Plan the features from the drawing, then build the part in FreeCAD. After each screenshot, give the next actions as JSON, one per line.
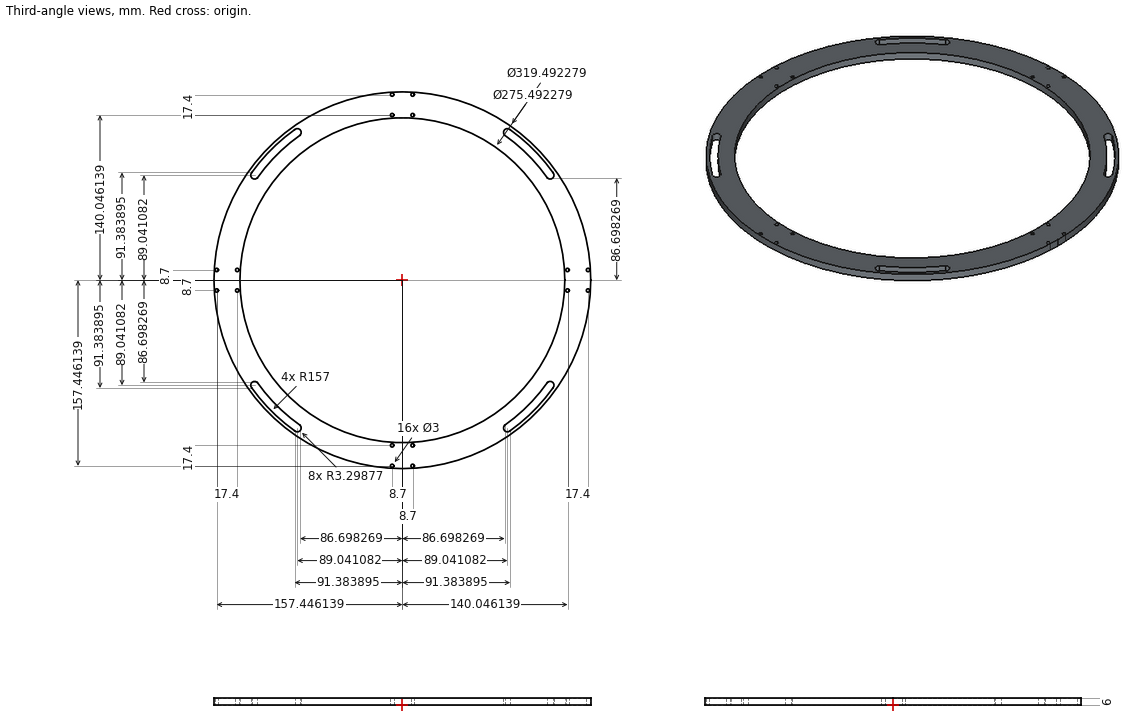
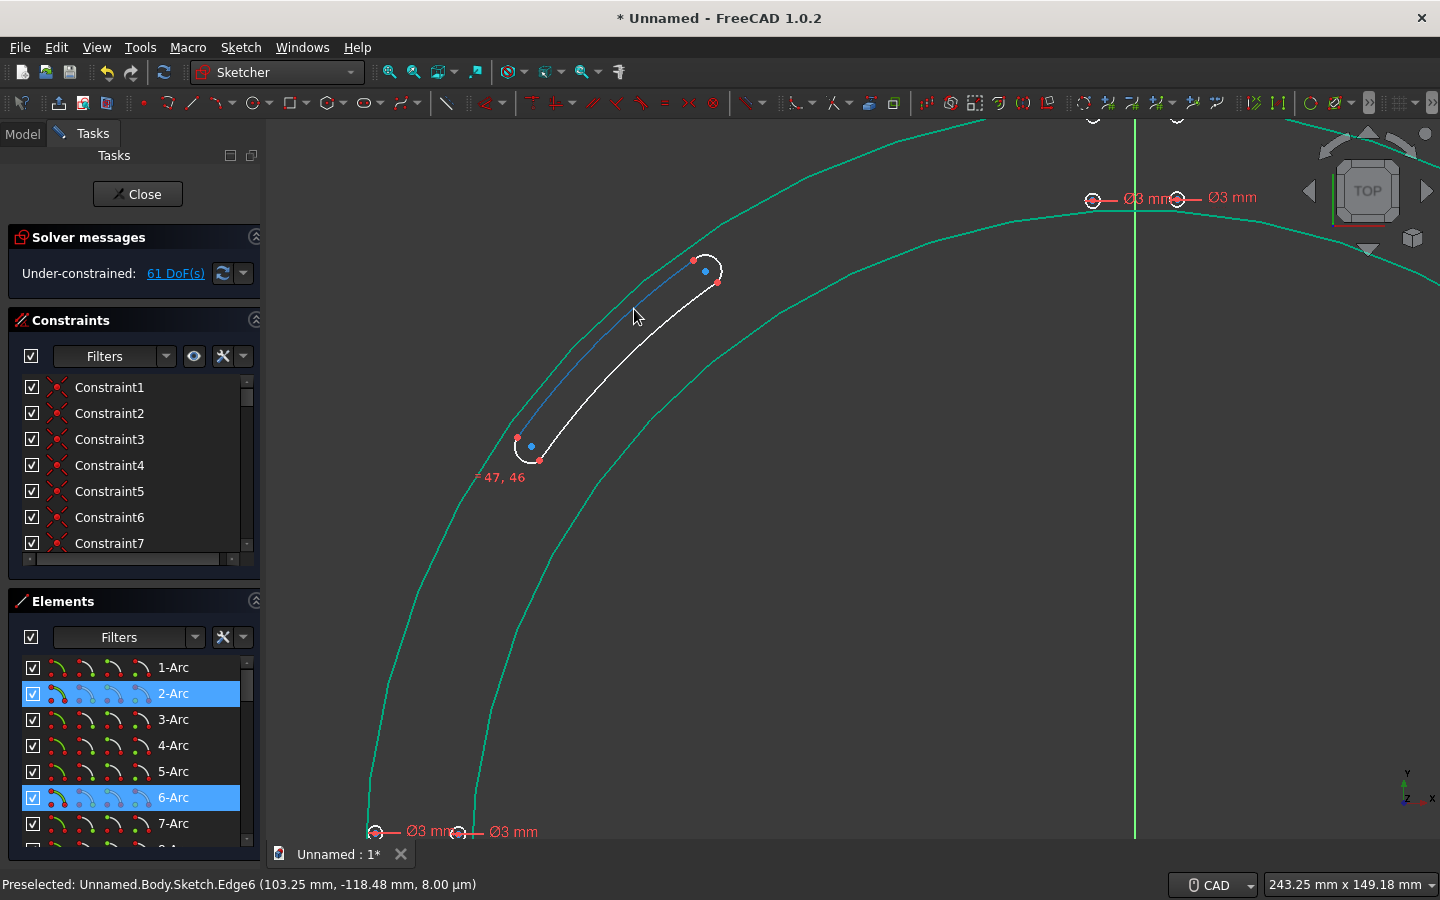
{"action": "left_click", "coordinate": [635, 307]}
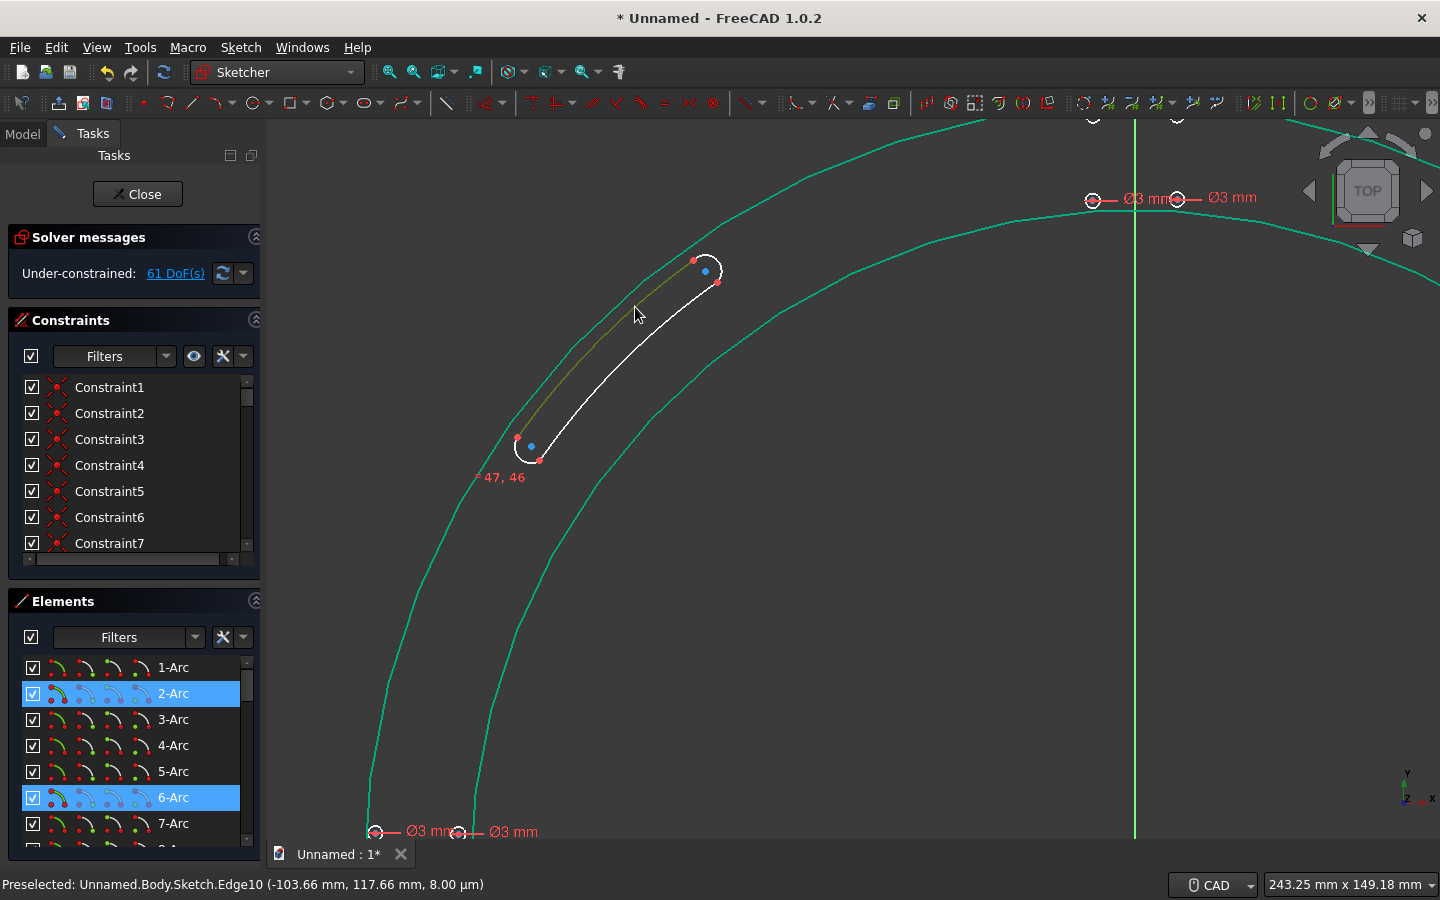
{"action": "scroll", "coordinate": [633, 308], "scroll_direction": "down", "scroll_amount": 6}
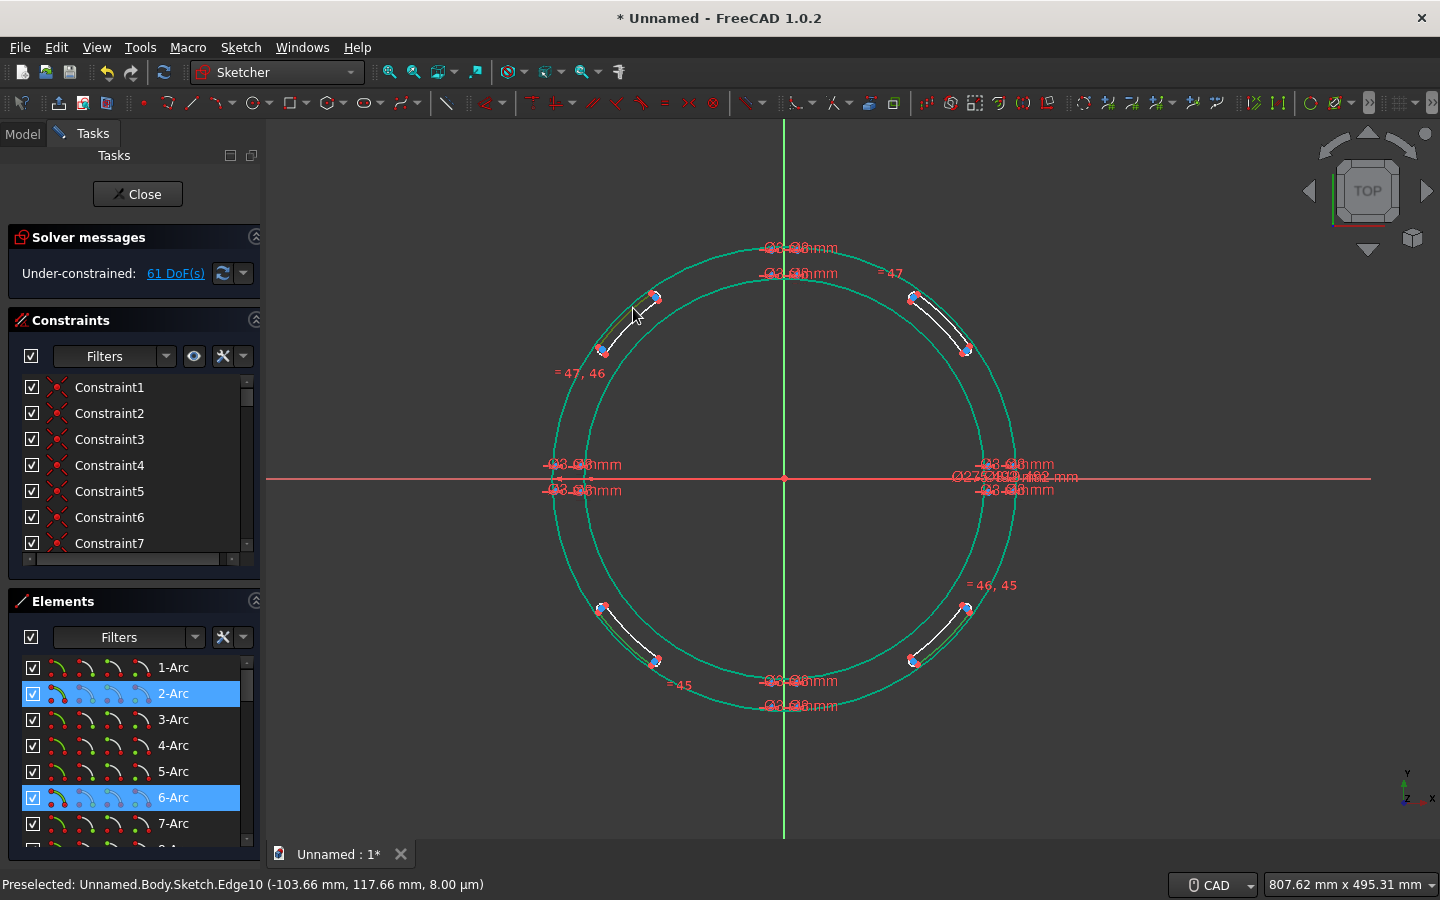
{"action": "scroll", "coordinate": [956, 329], "scroll_direction": "up", "scroll_amount": 6}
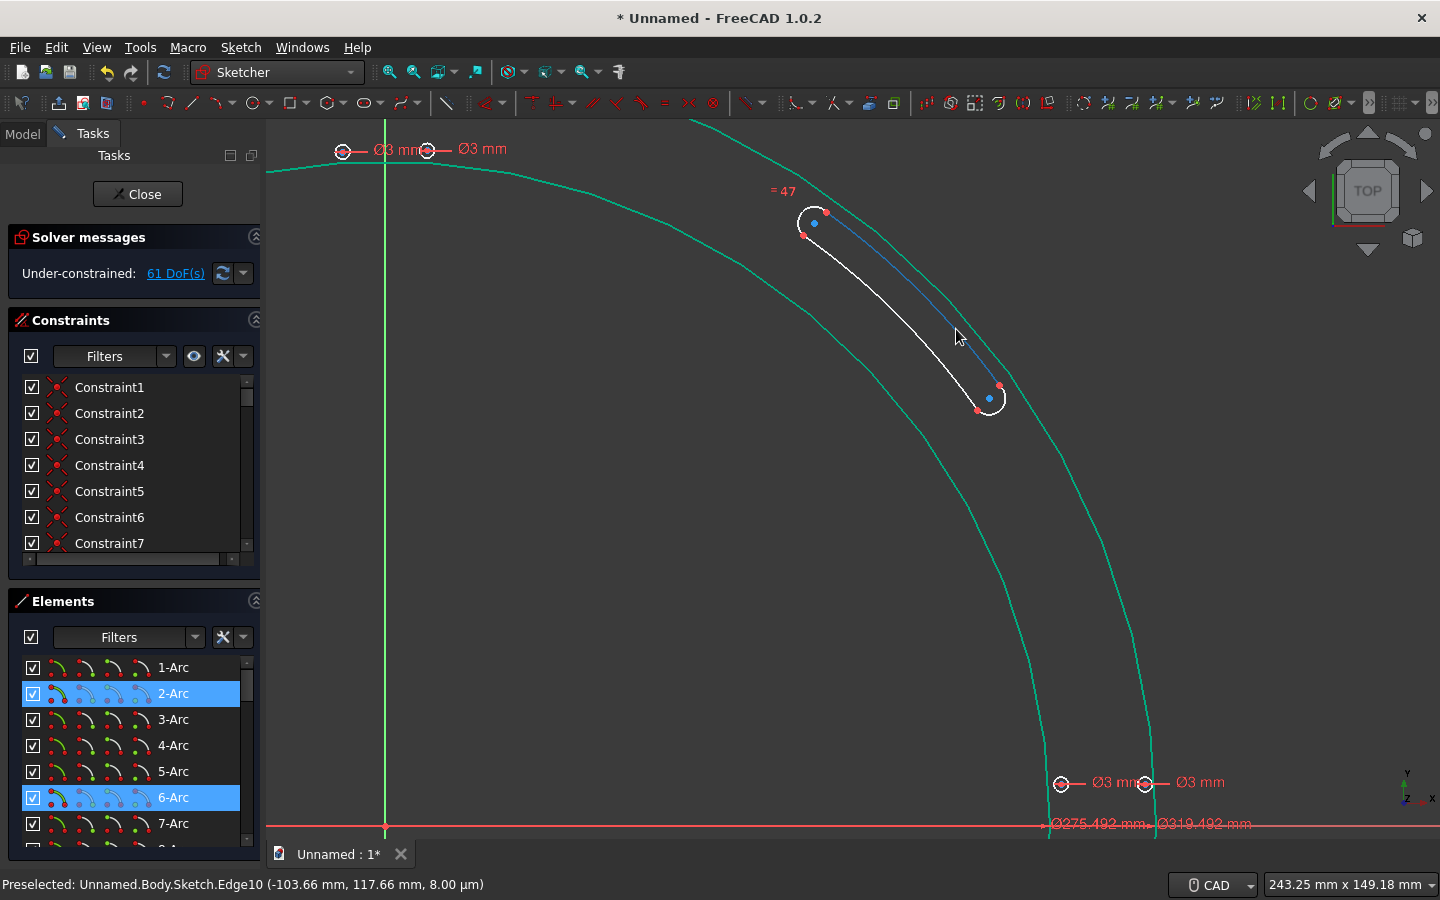
{"action": "left_click", "coordinate": [954, 328]}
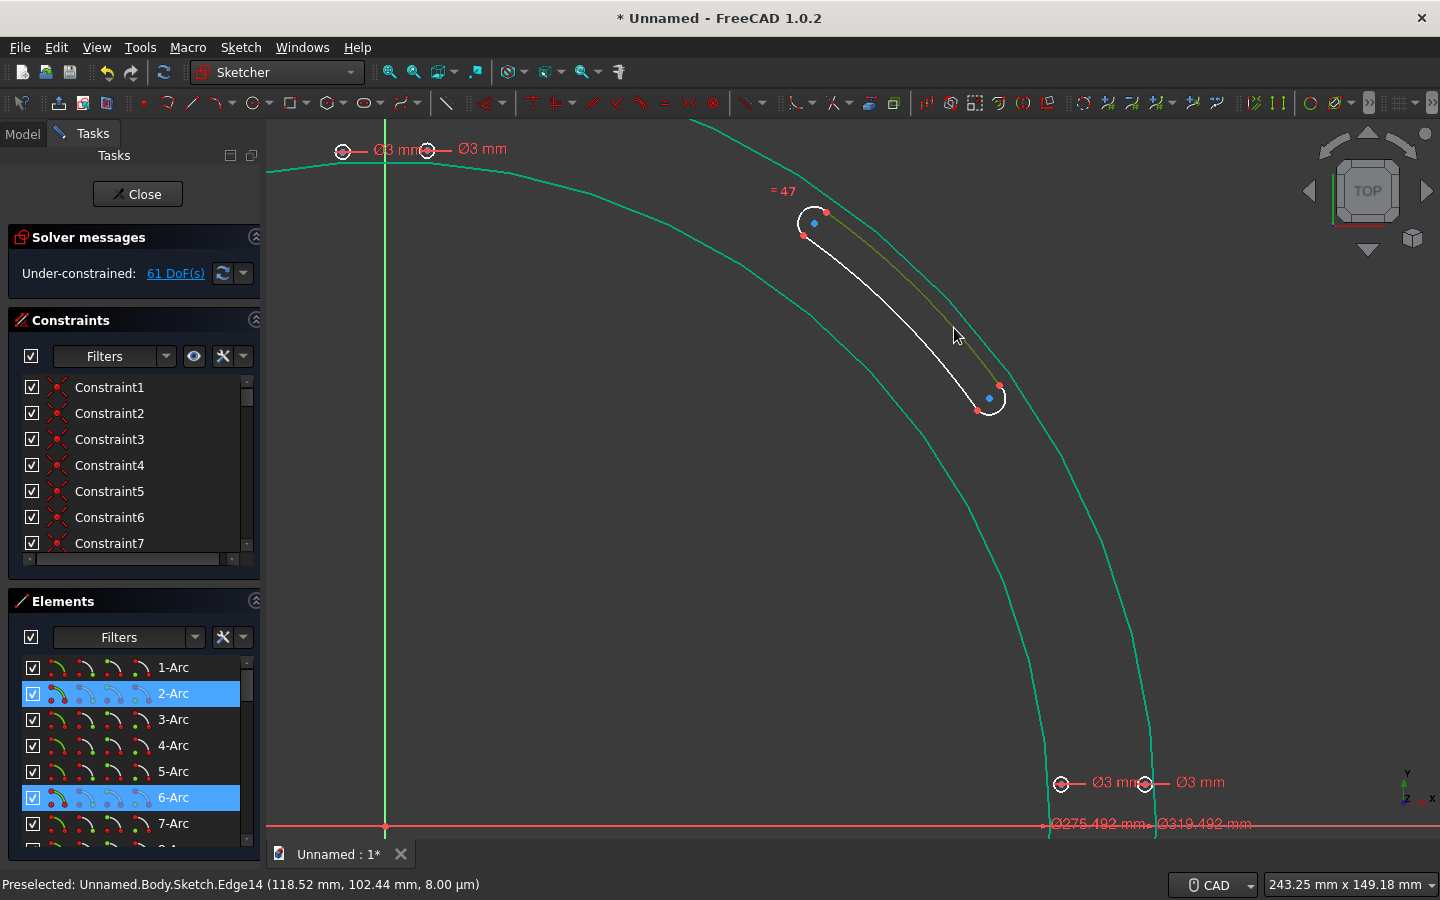
{"action": "key", "text": "e"}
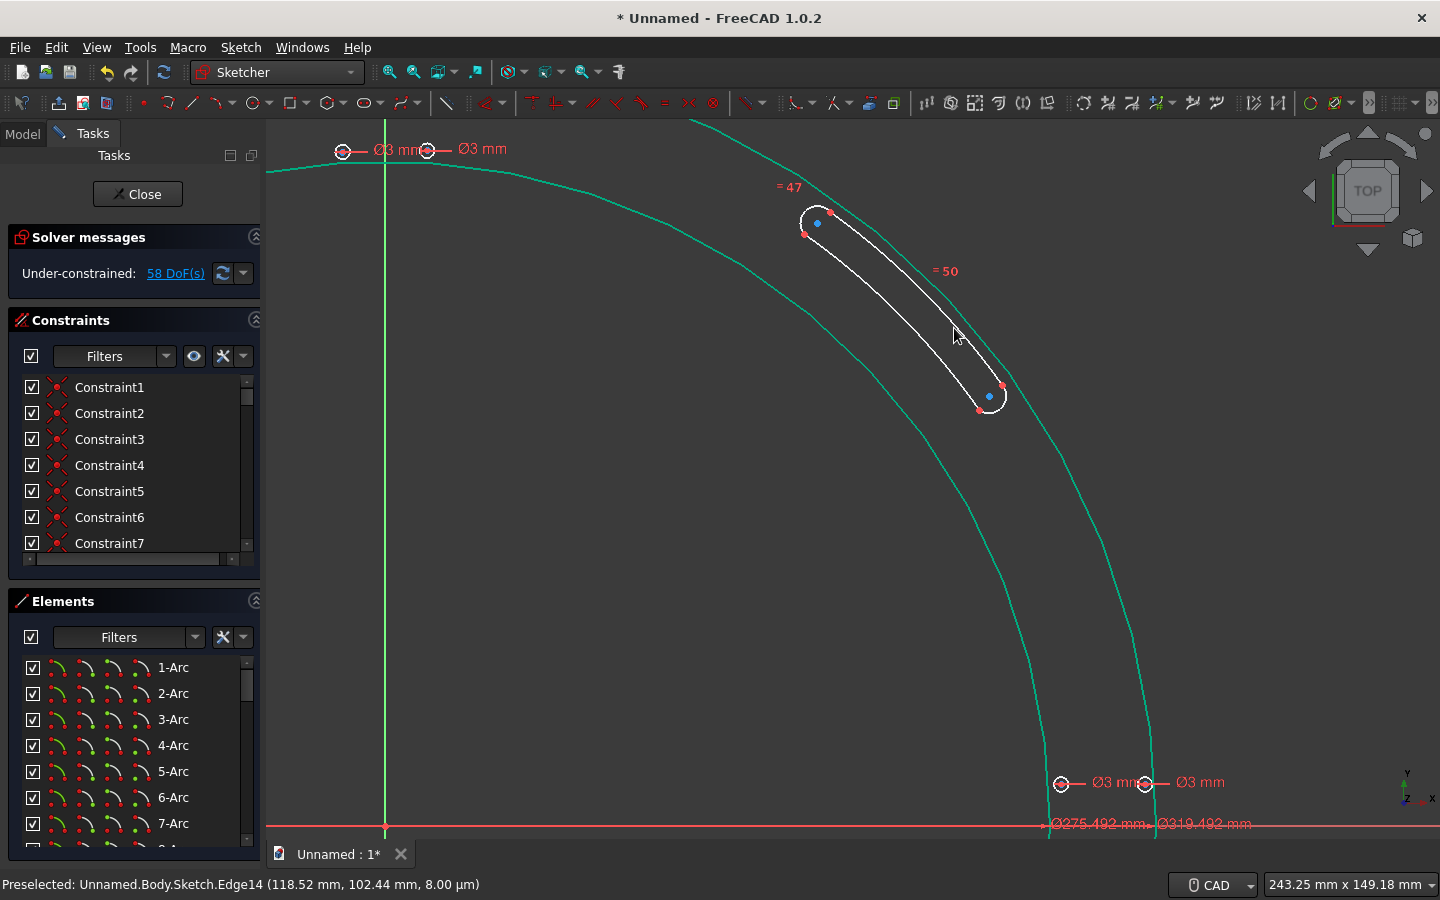
{"action": "scroll", "coordinate": [957, 329], "scroll_direction": "down", "scroll_amount": 6}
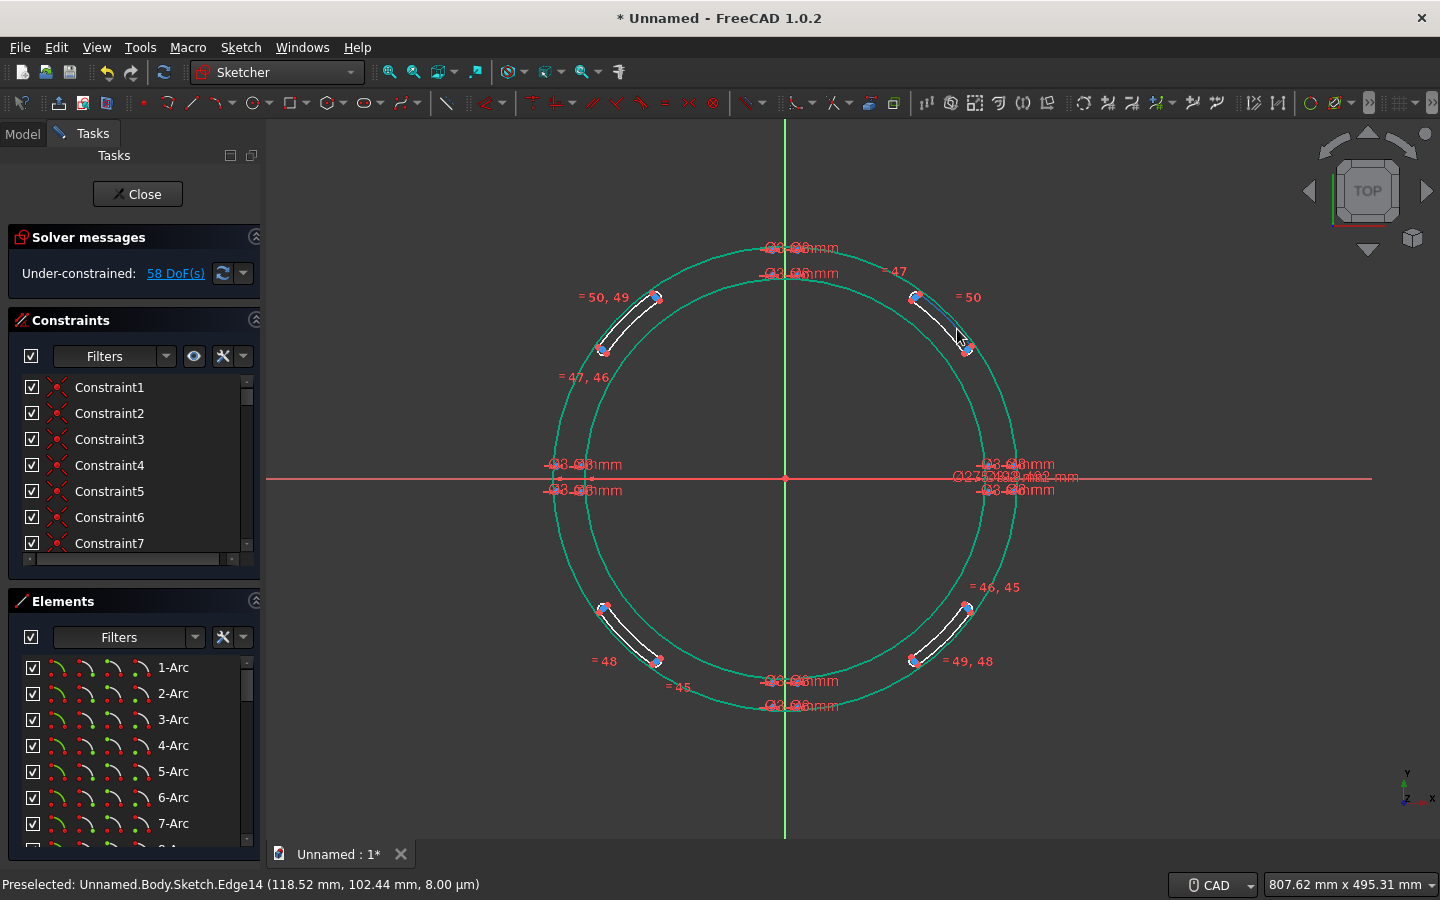
{"action": "scroll", "coordinate": [621, 623], "scroll_direction": "up", "scroll_amount": 2}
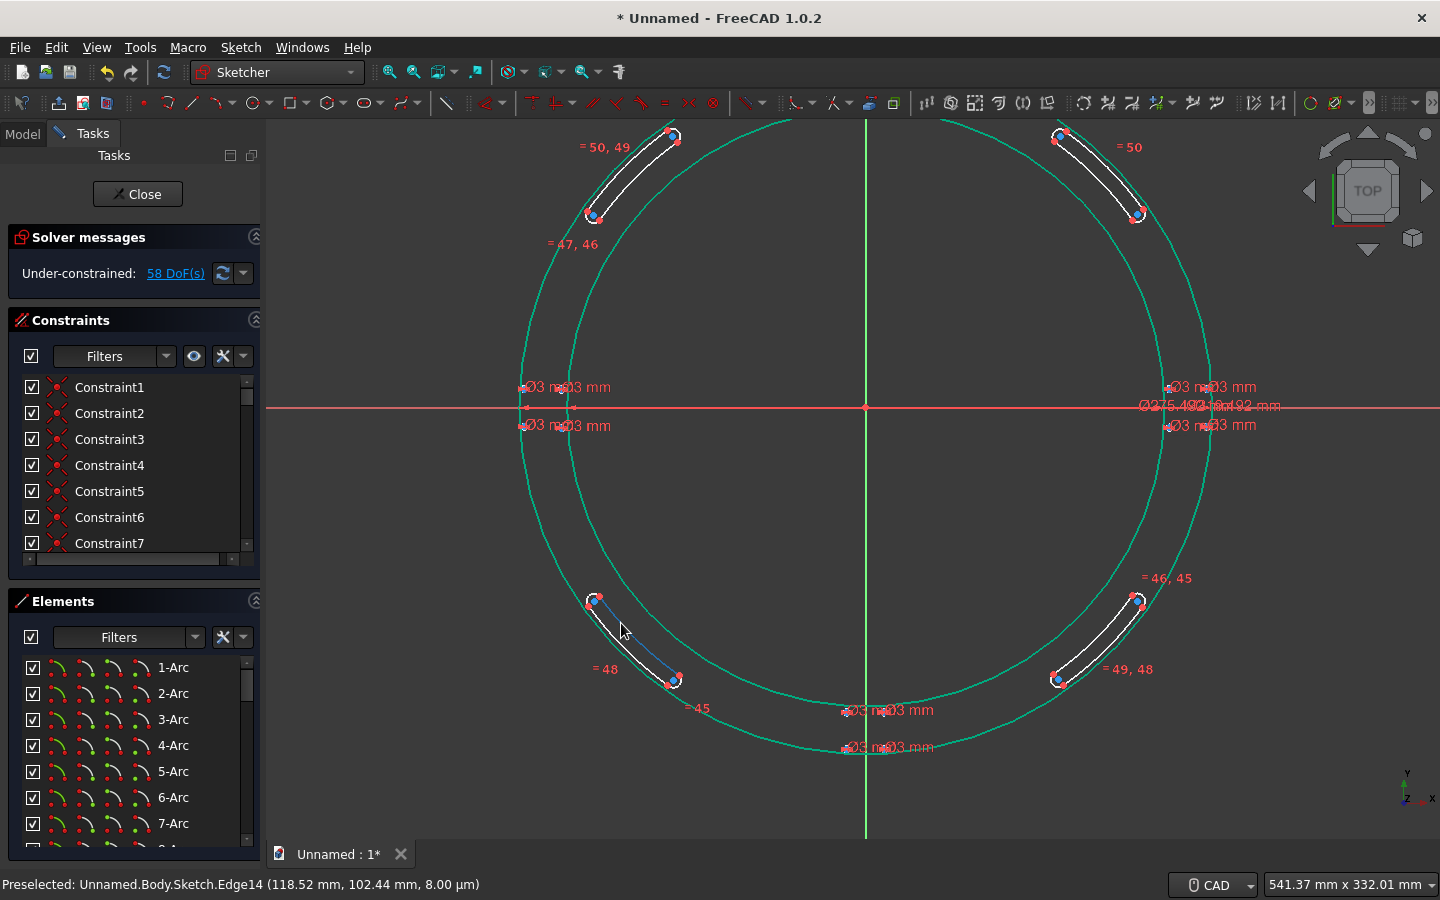
{"action": "left_click", "coordinate": [621, 623]}